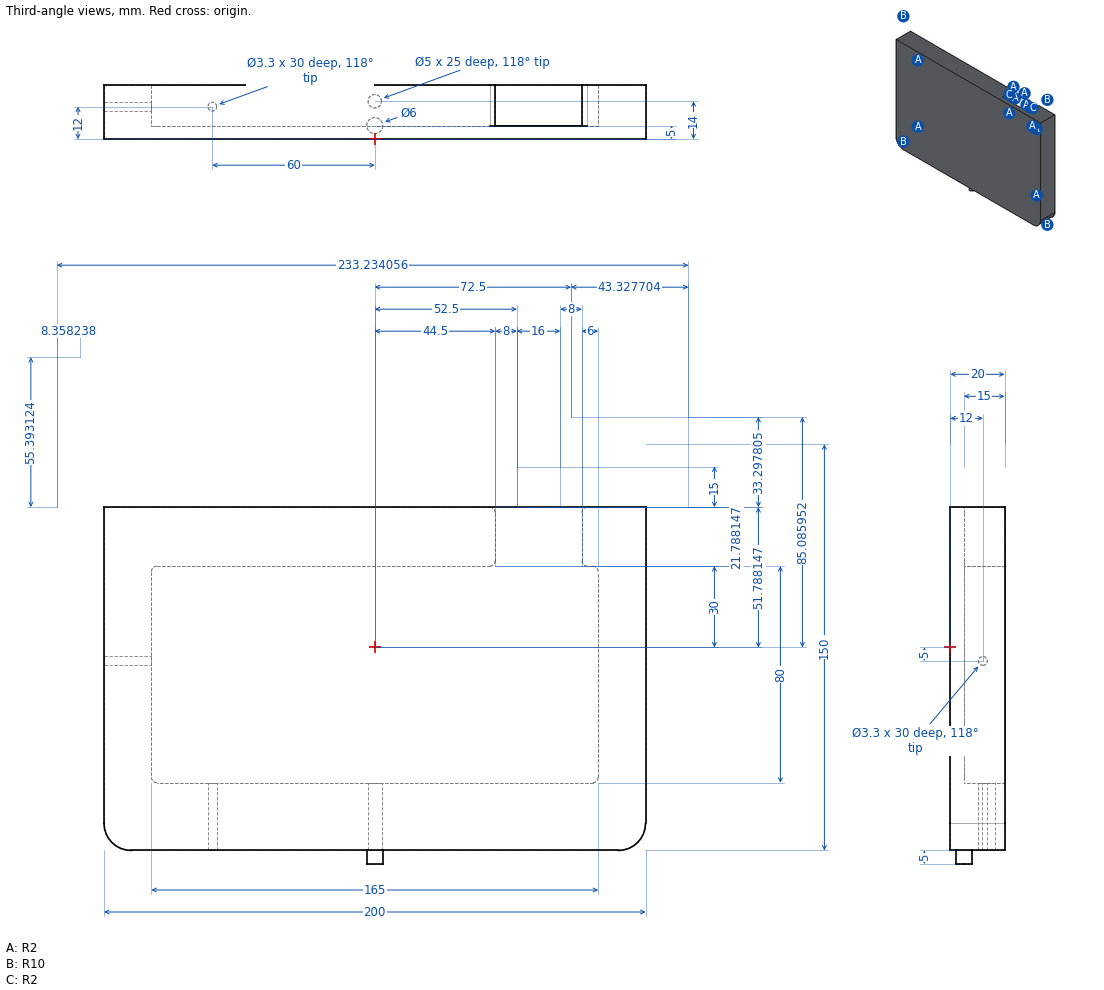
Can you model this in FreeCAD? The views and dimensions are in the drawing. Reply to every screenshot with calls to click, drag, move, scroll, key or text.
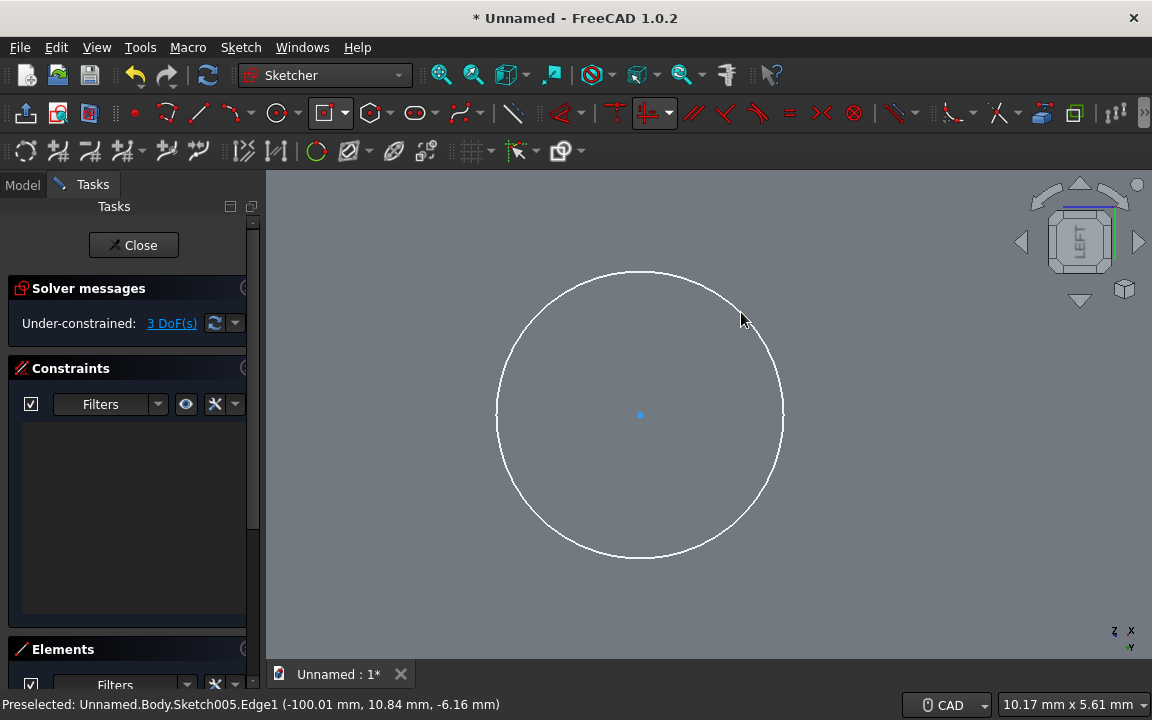
click(560, 114)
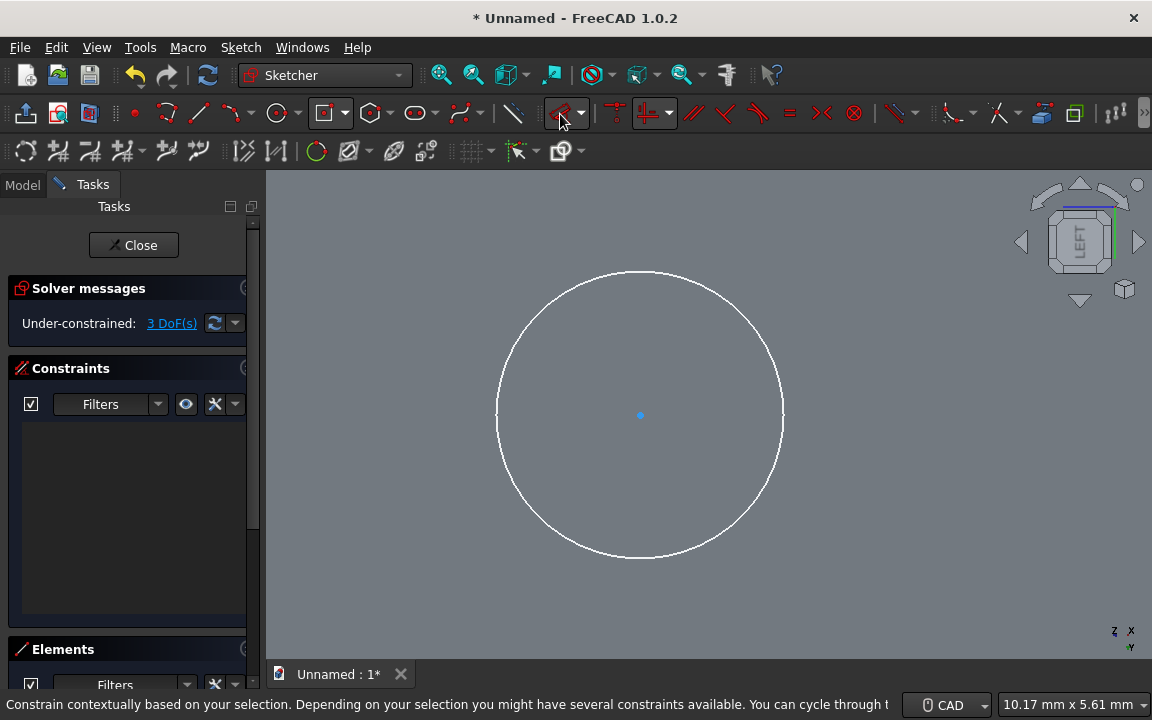
click(741, 313)
click(764, 290)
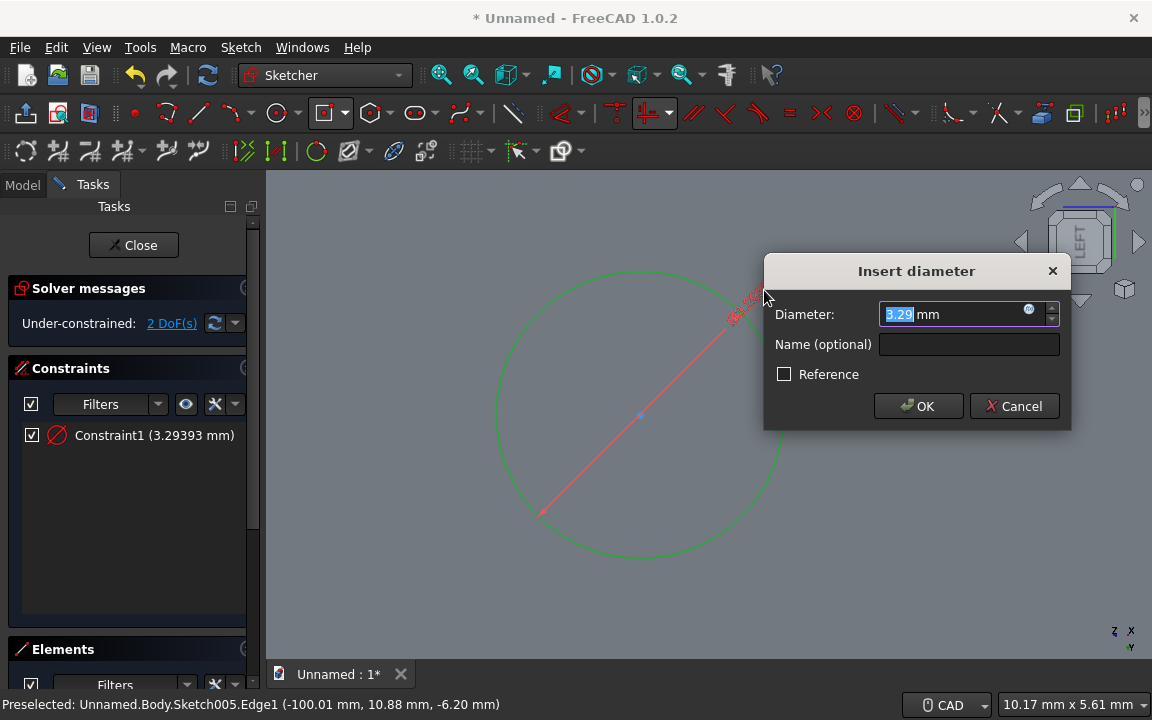
text(3.3)
key(Return)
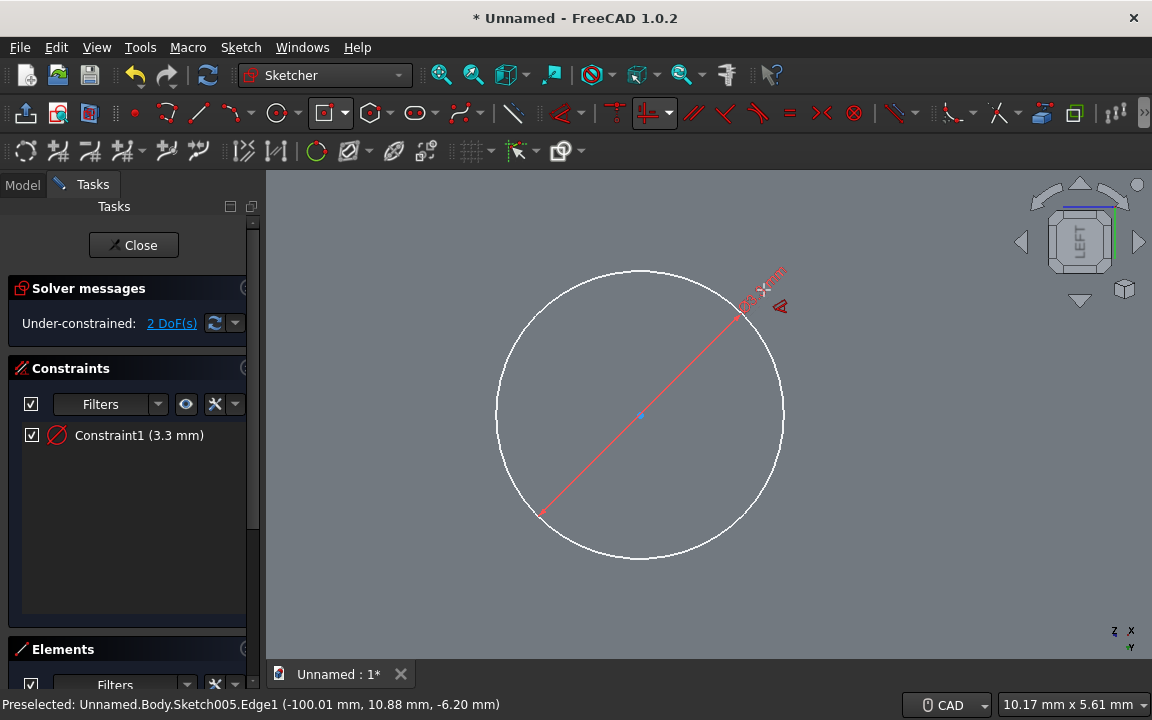
click(640, 415)
click(467, 449)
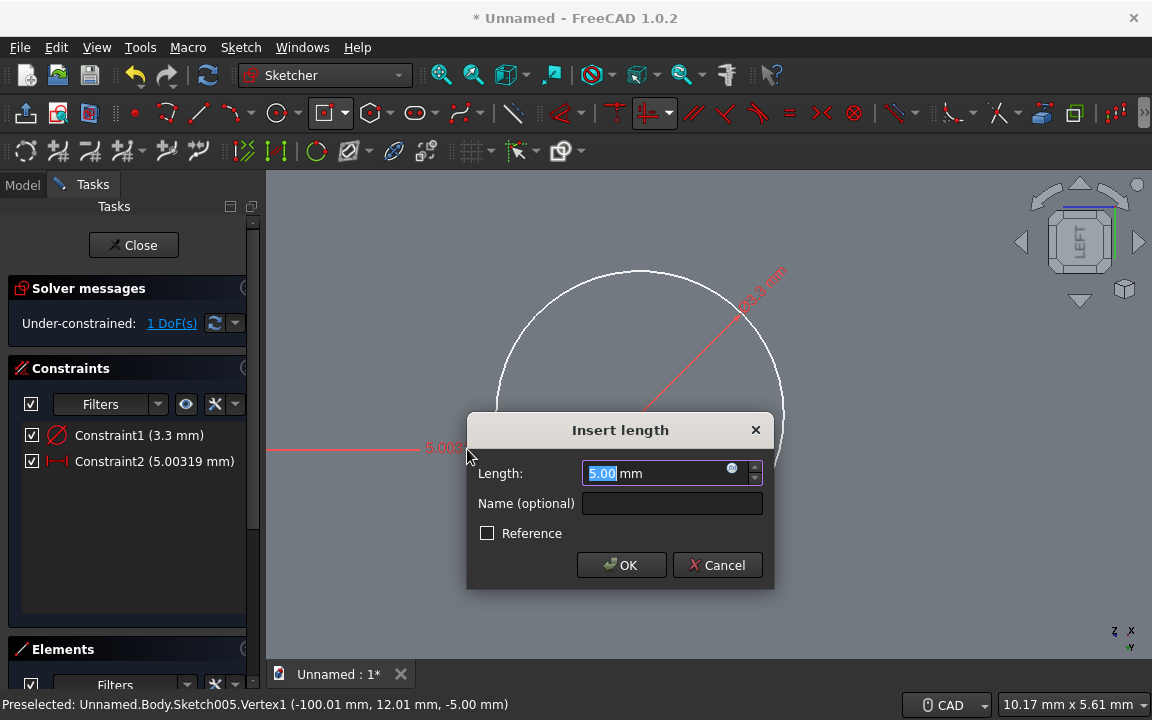
text(5)
key(Return)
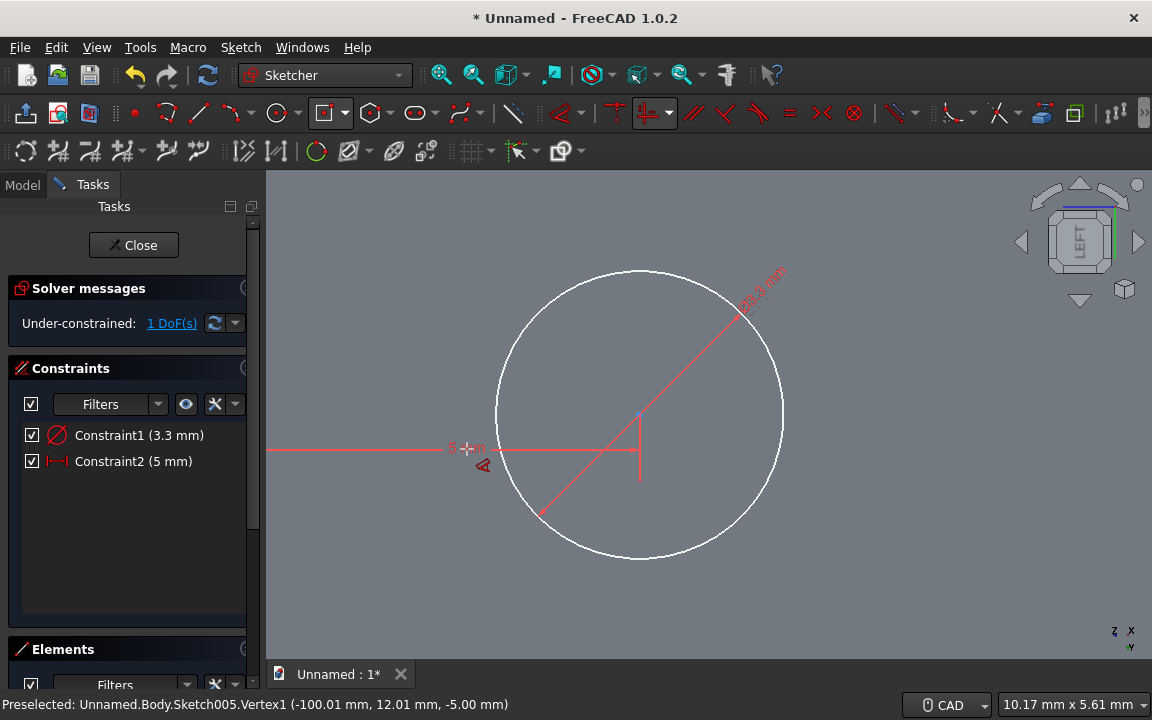
click(640, 415)
click(674, 306)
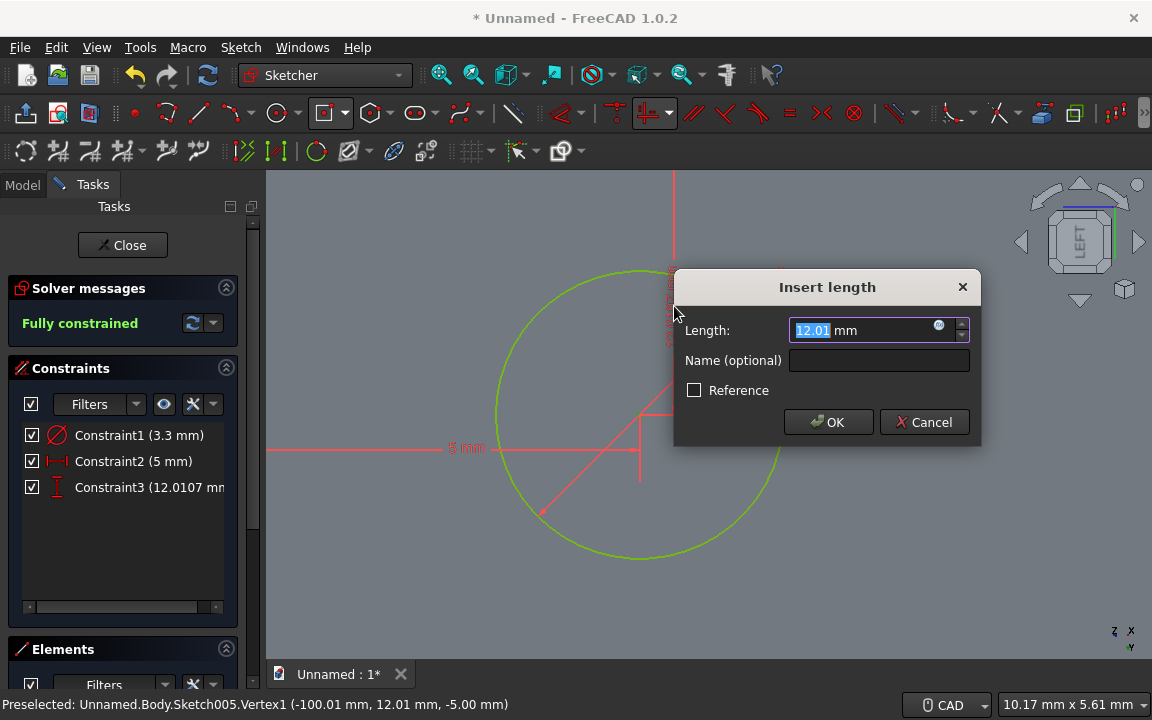
text(12)
key(Return)
key(Escape)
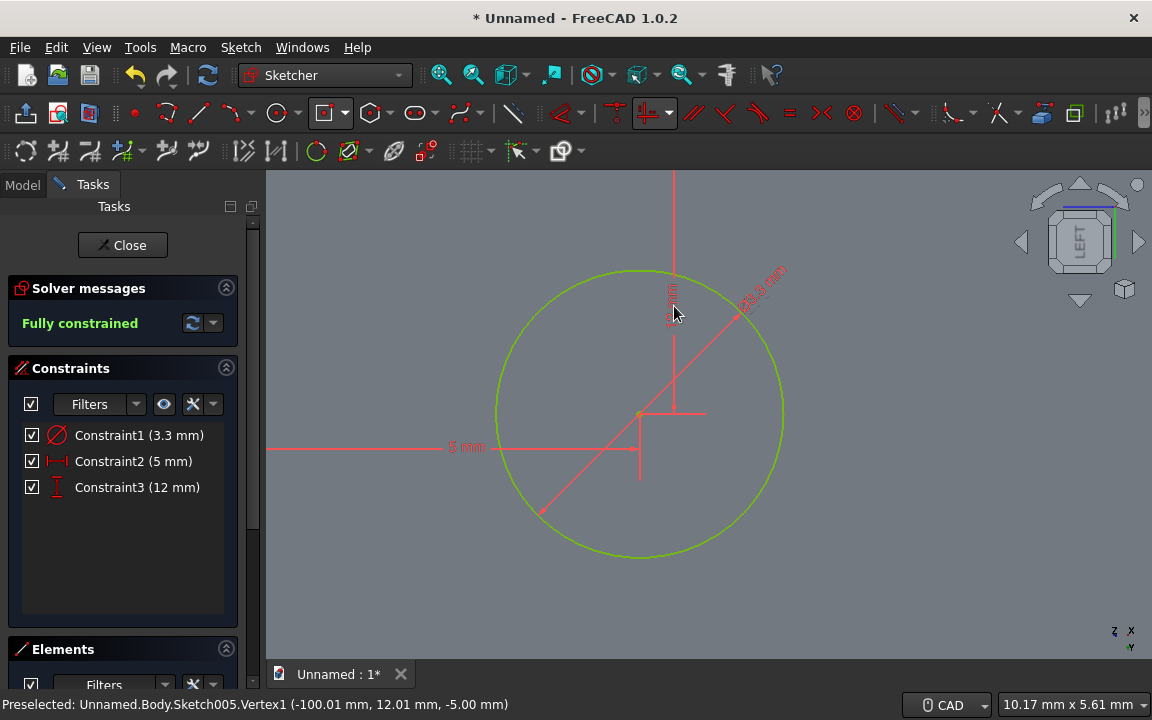
click(123, 245)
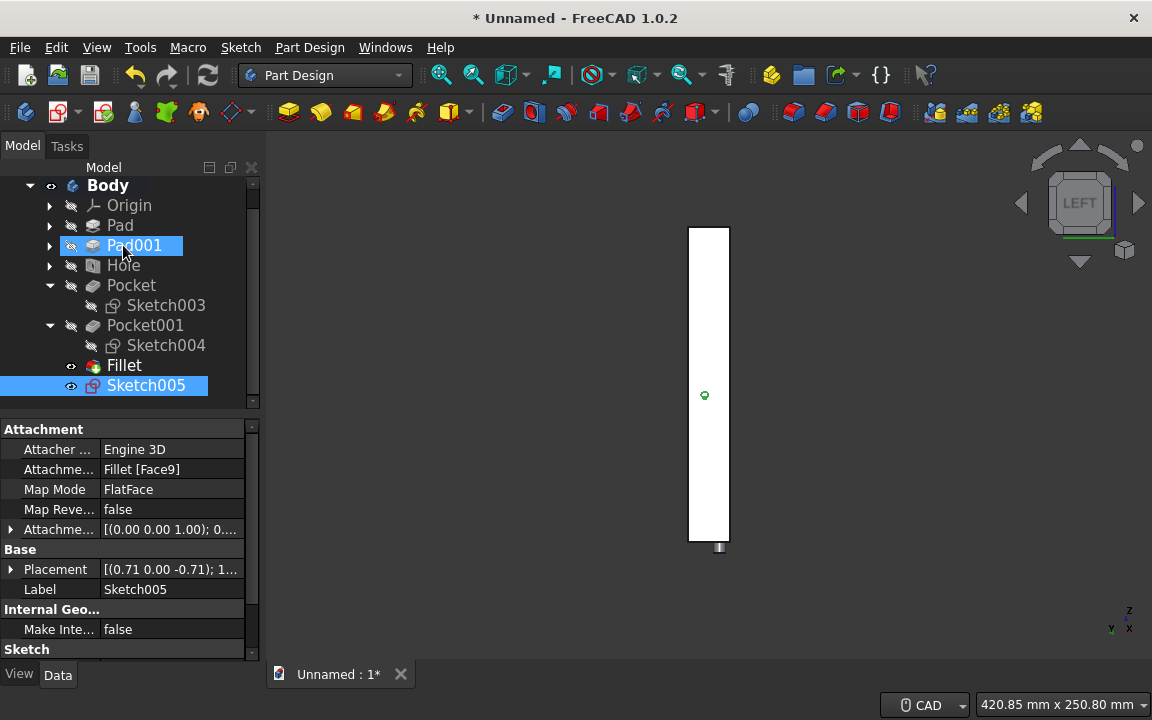
click(536, 112)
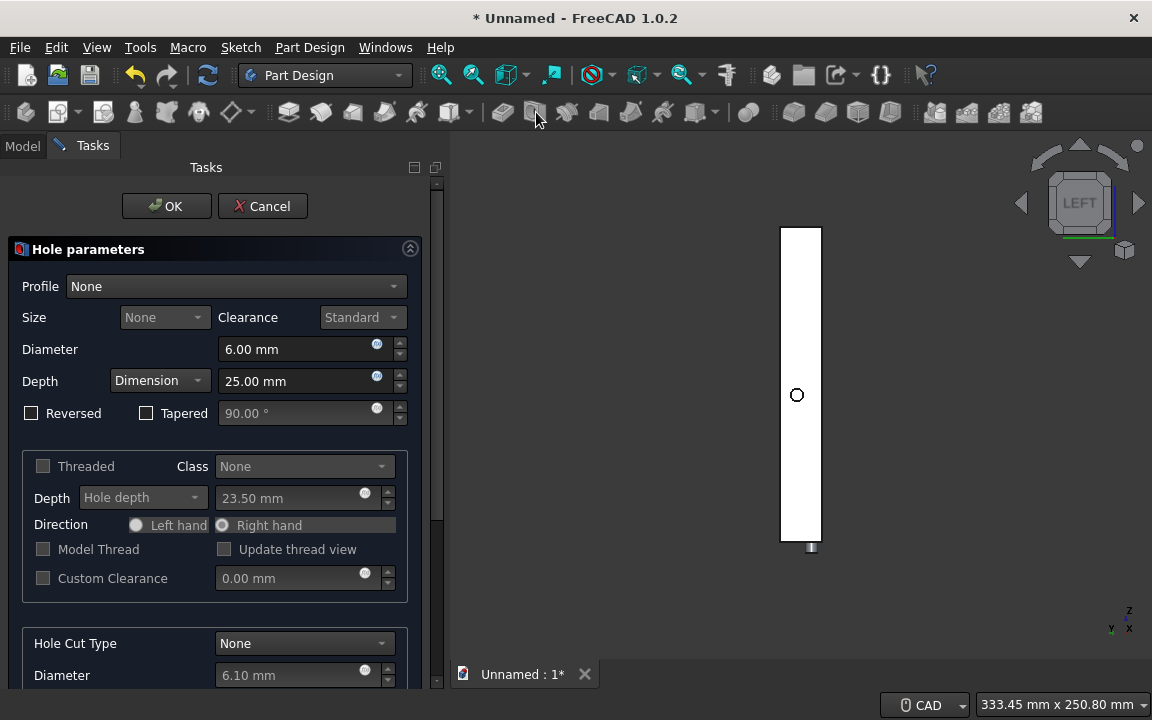
triple_click(305, 349)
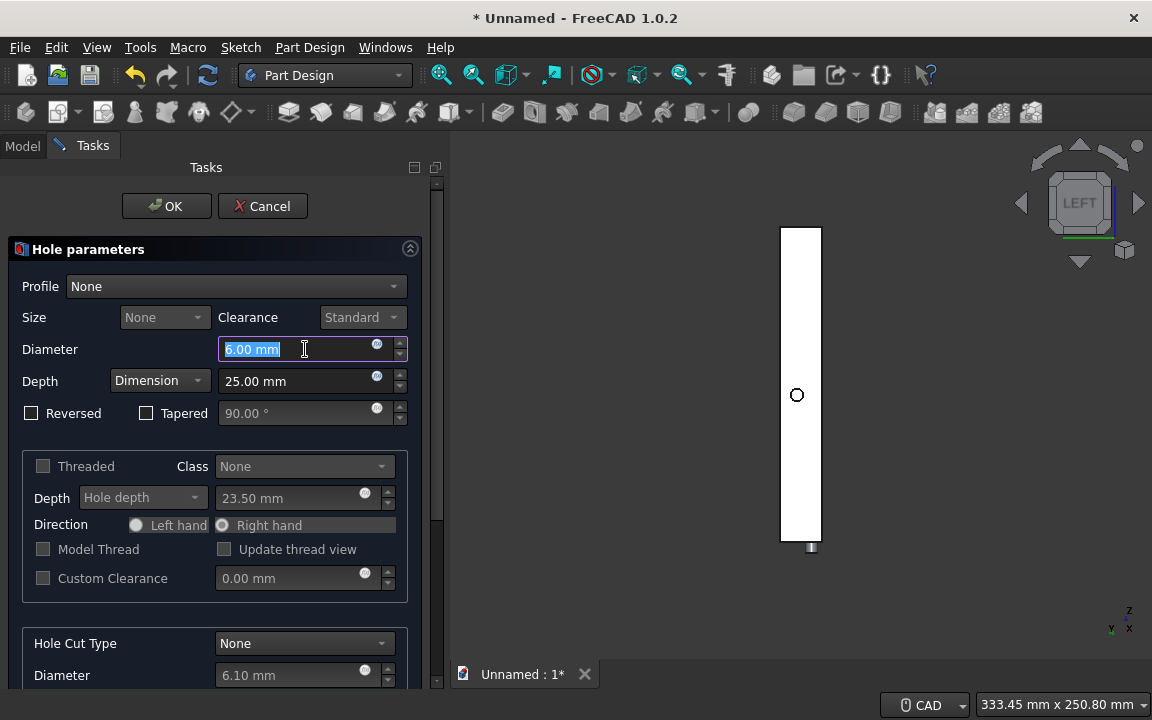
text(3.3)
key(Tab)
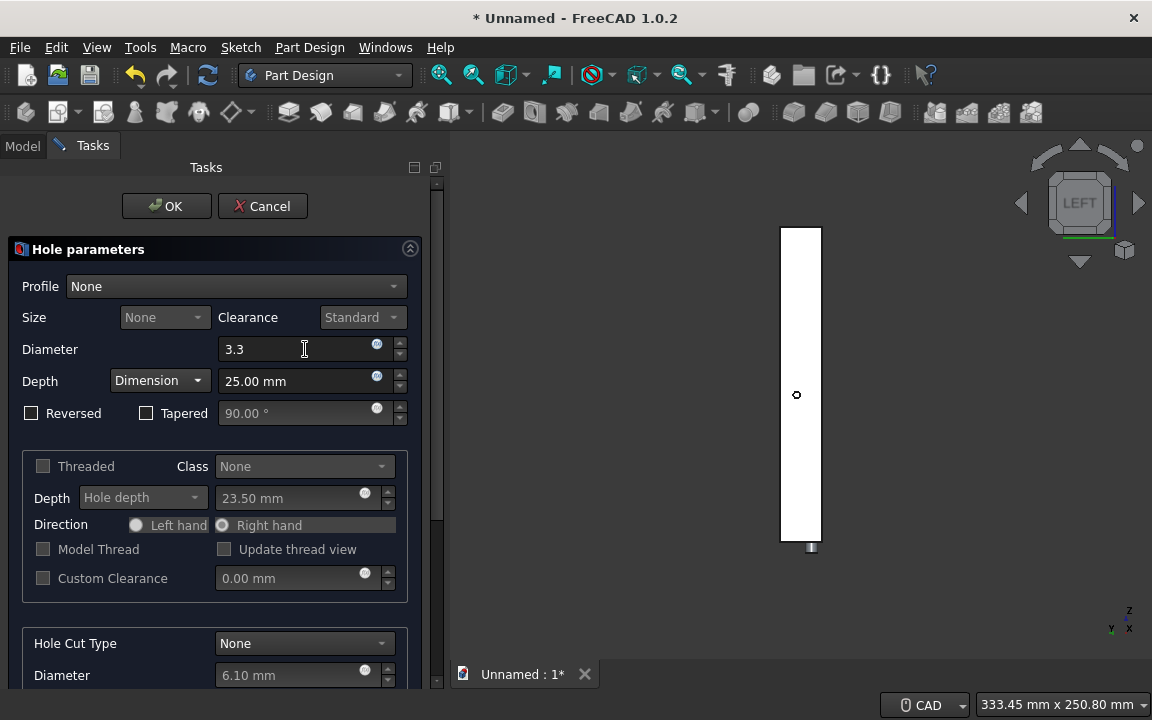
triple_click(305, 381)